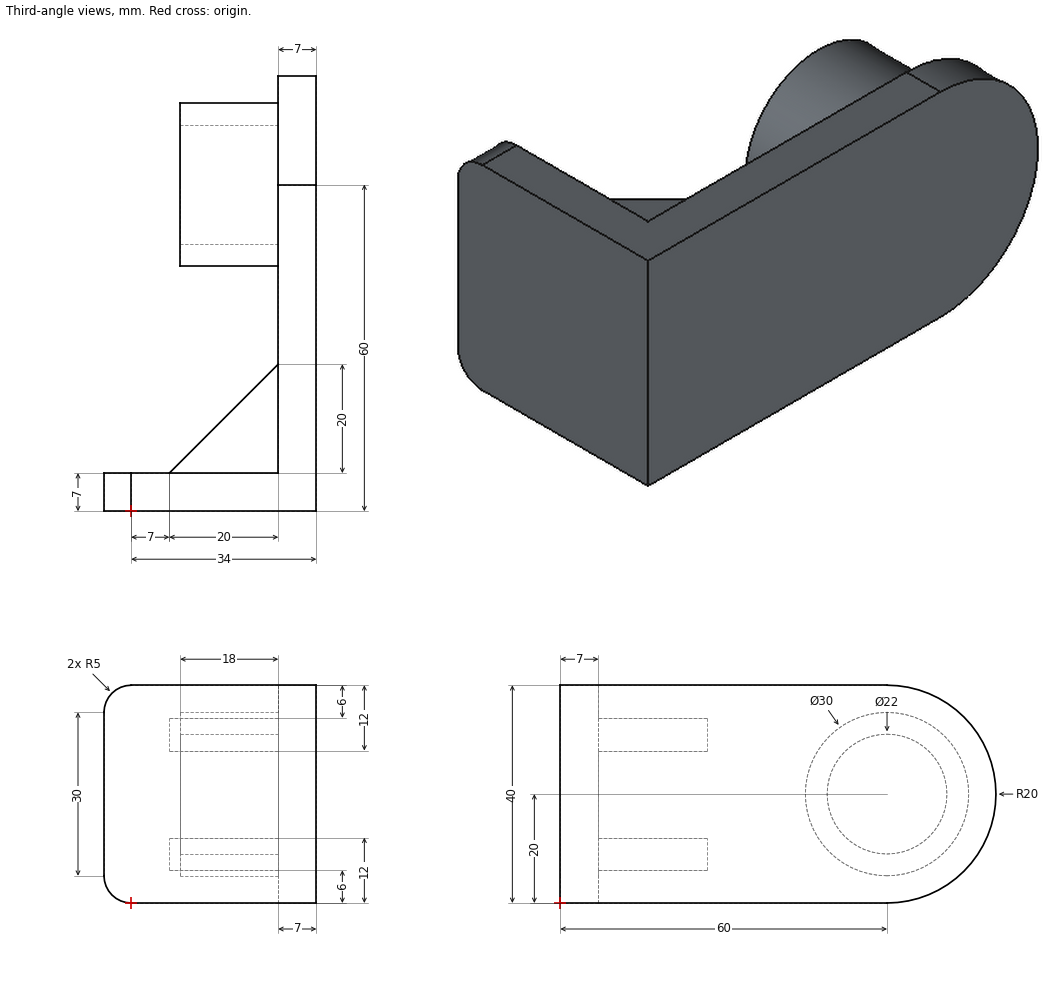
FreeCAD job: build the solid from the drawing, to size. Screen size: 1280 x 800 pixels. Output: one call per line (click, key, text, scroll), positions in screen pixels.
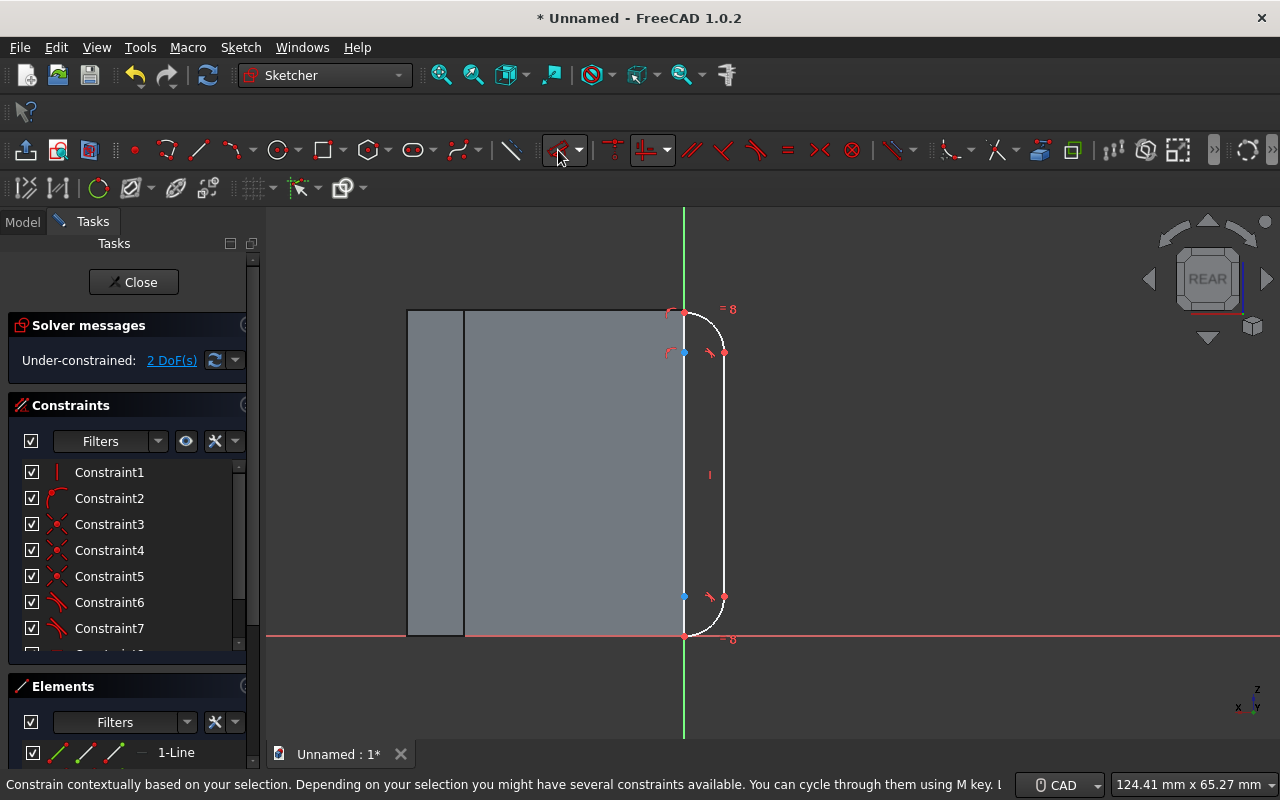
click(720, 334)
click(748, 319)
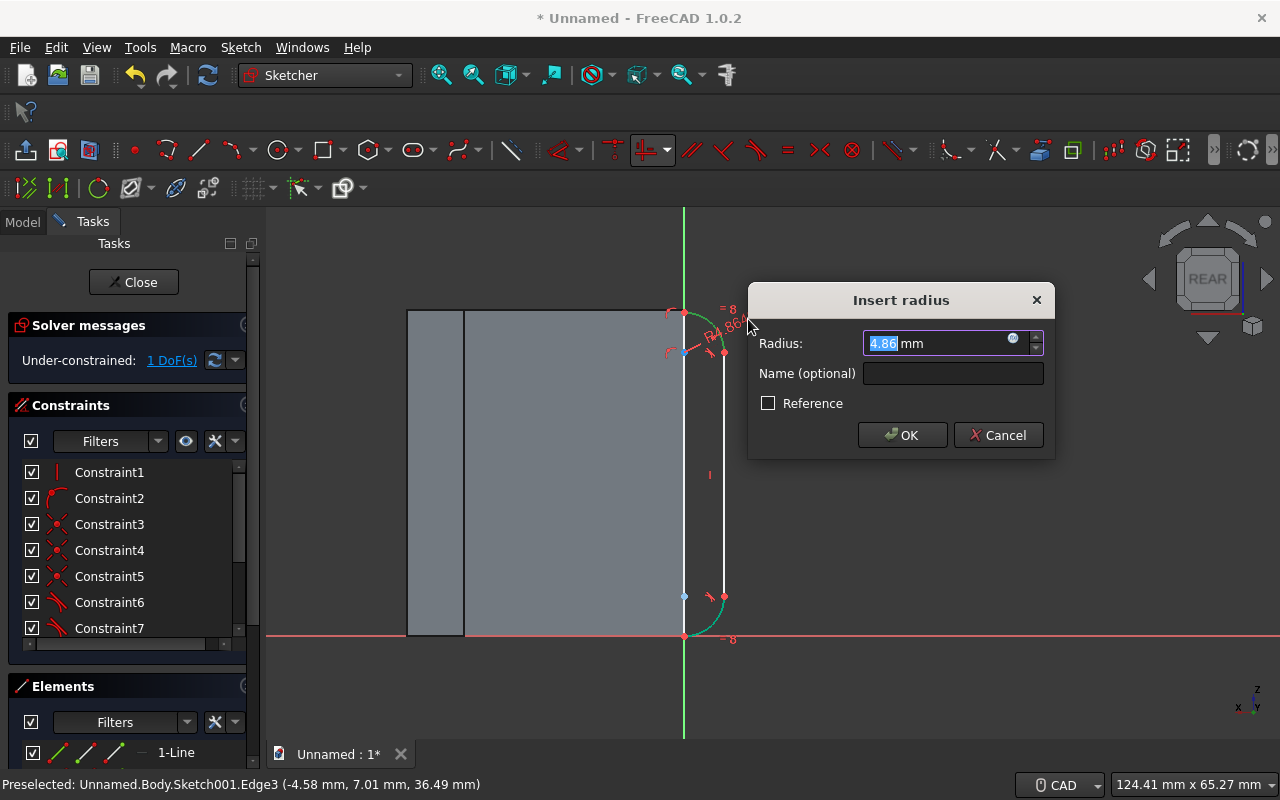
text(5)
key(Return)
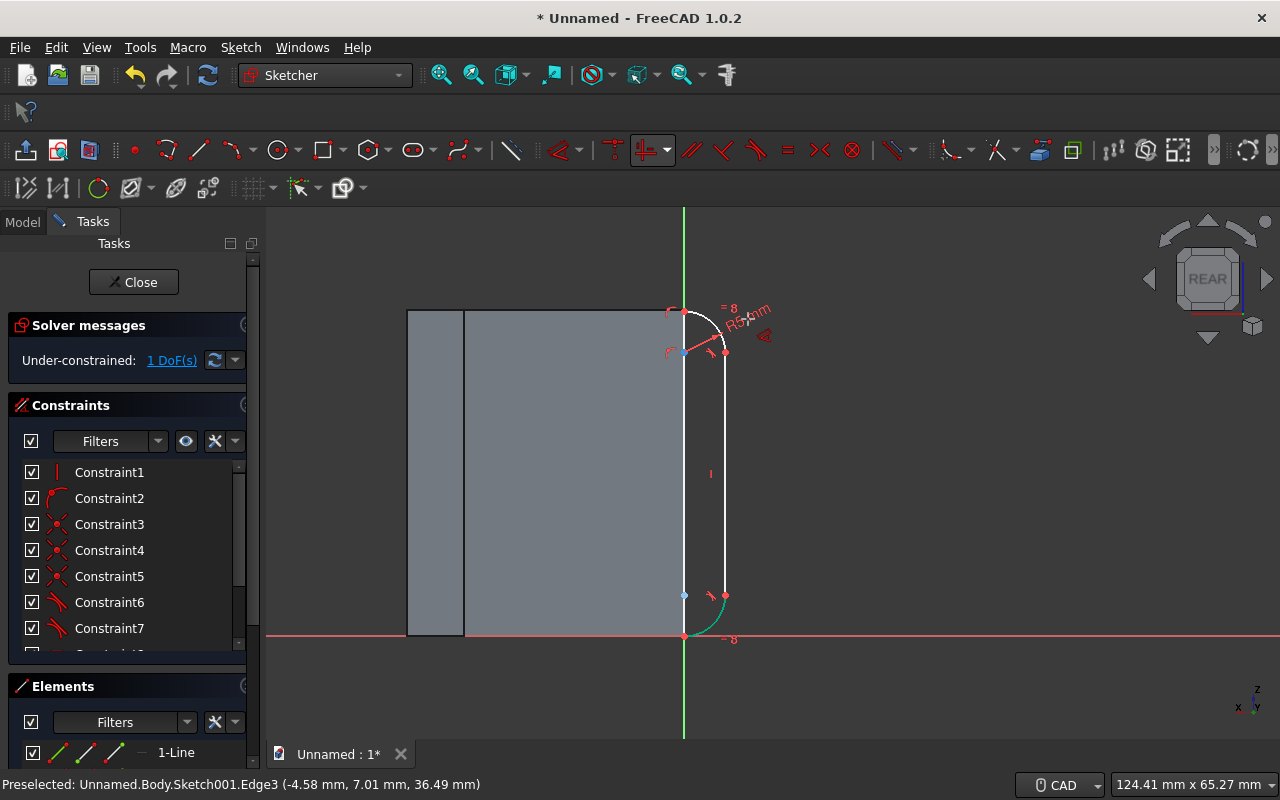
click(725, 523)
click(759, 474)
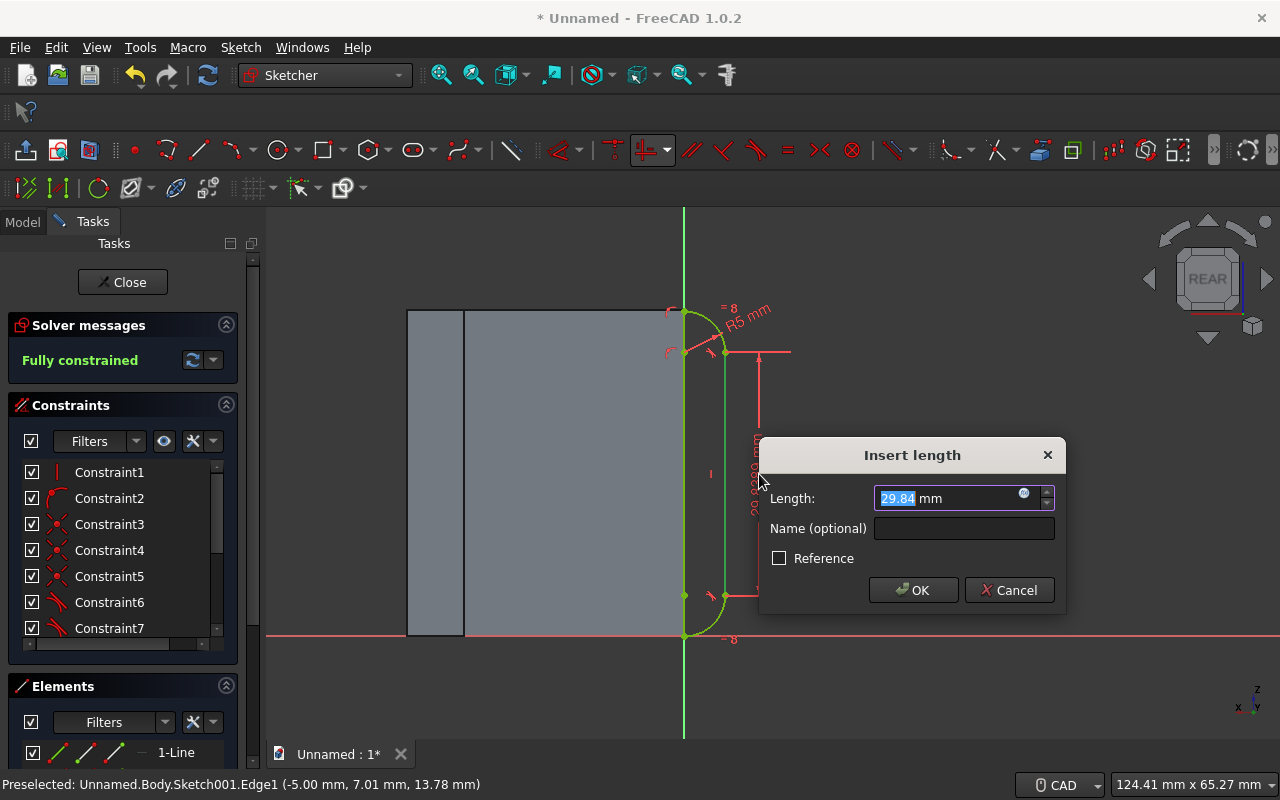
text(30)
key(Return)
key(Escape)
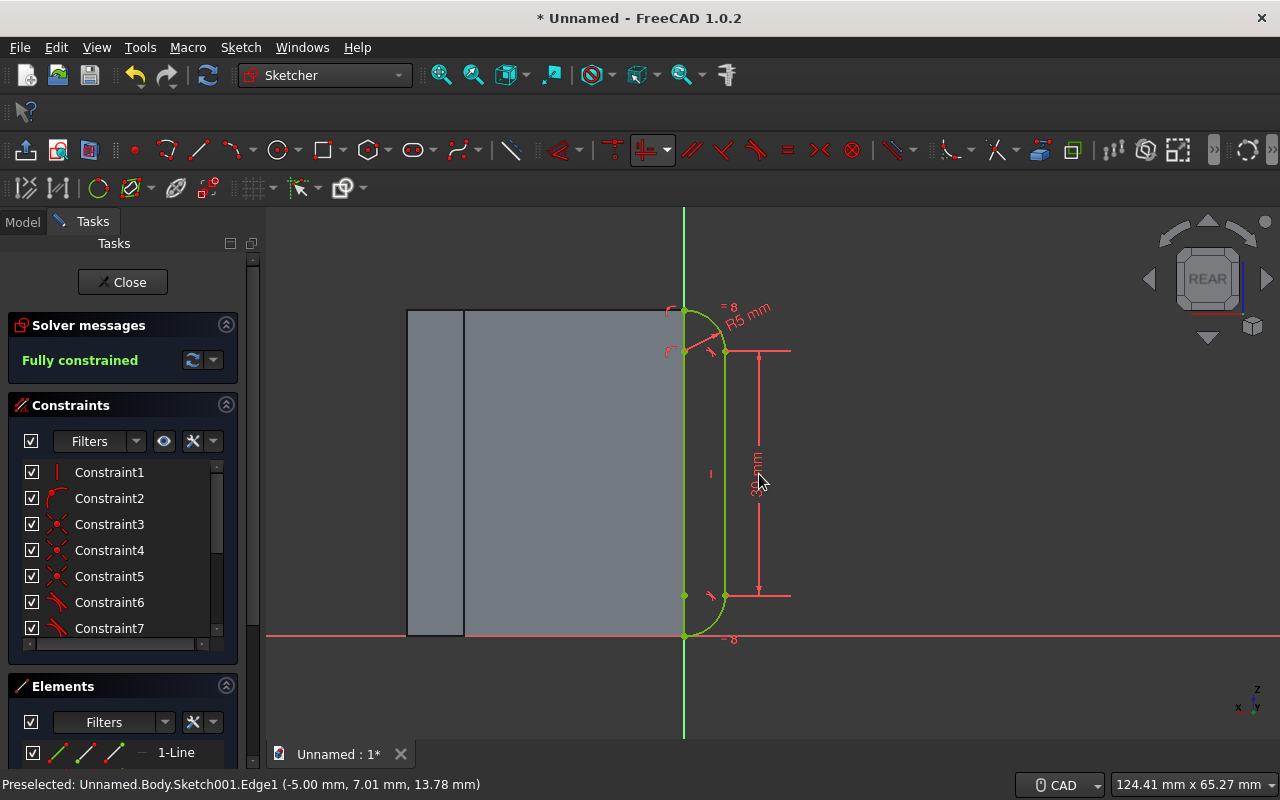
click(123, 282)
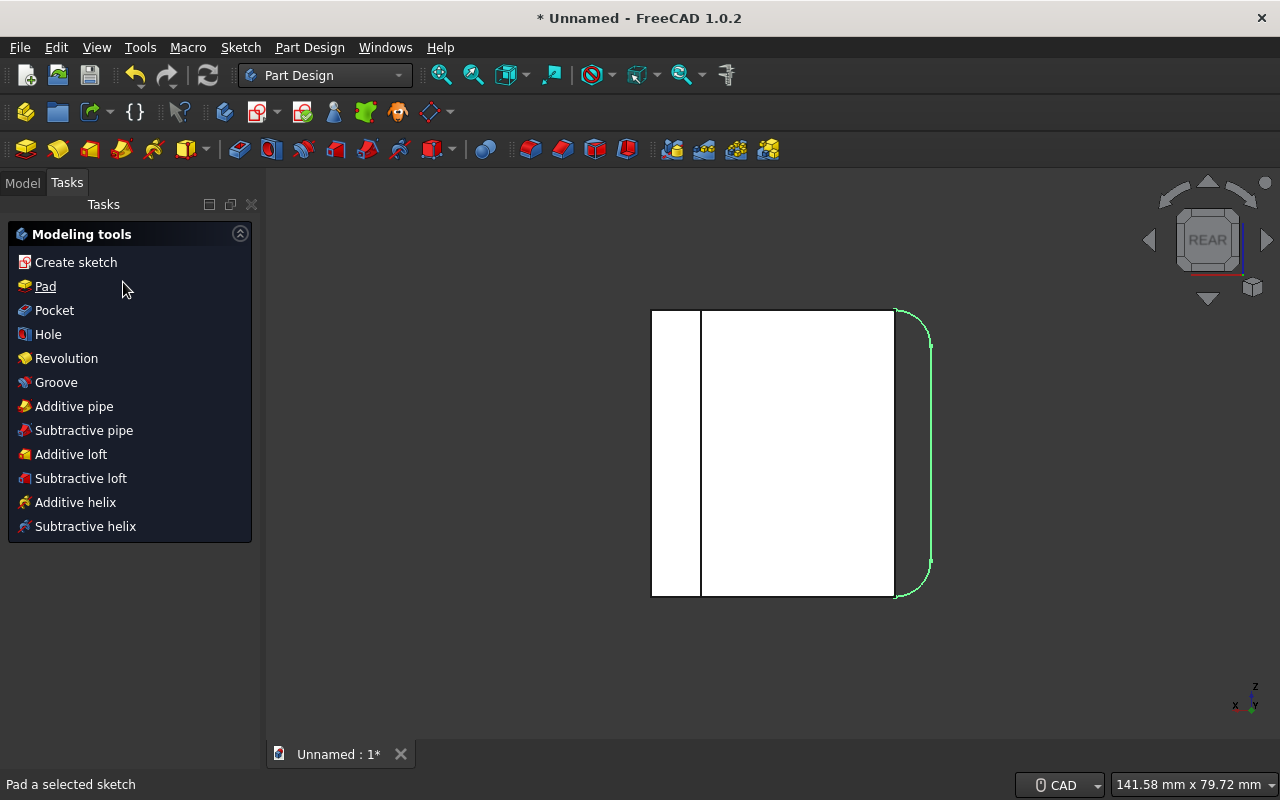
click(26, 150)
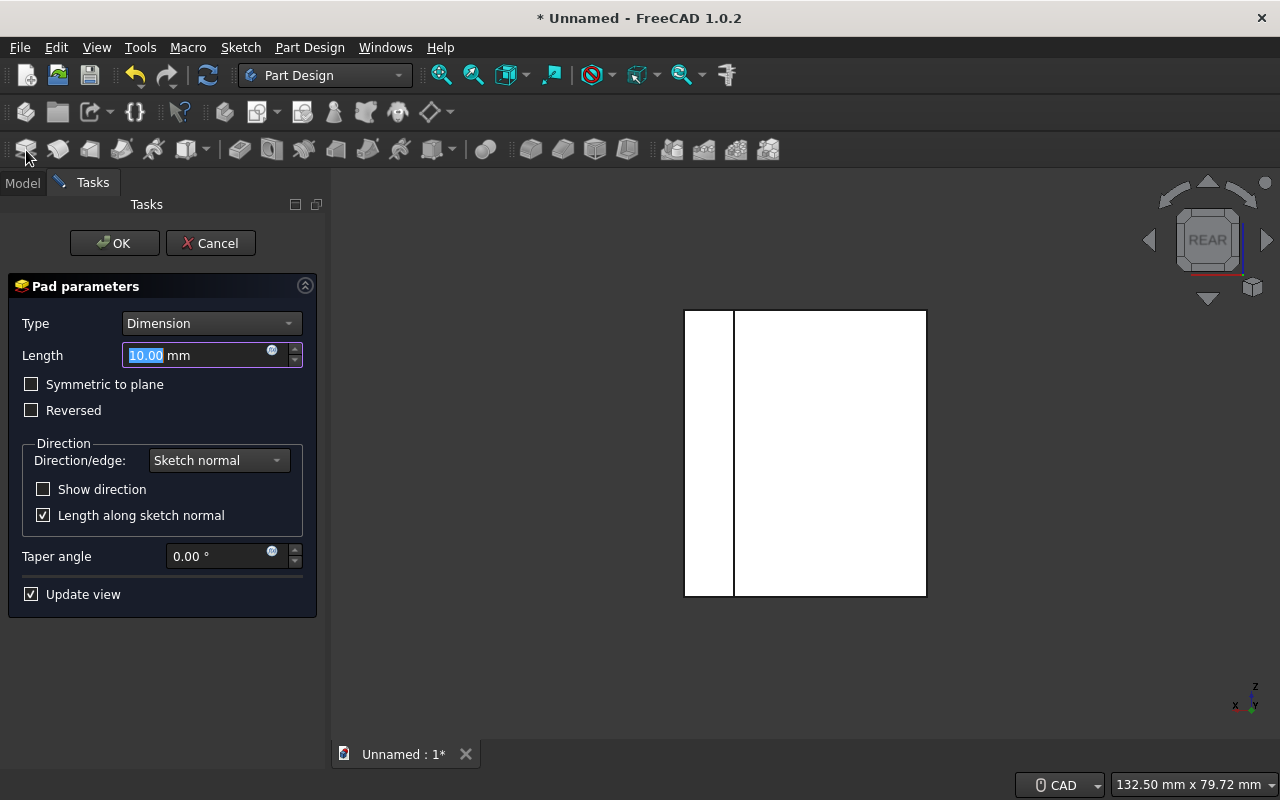
text(7)
key(Tab)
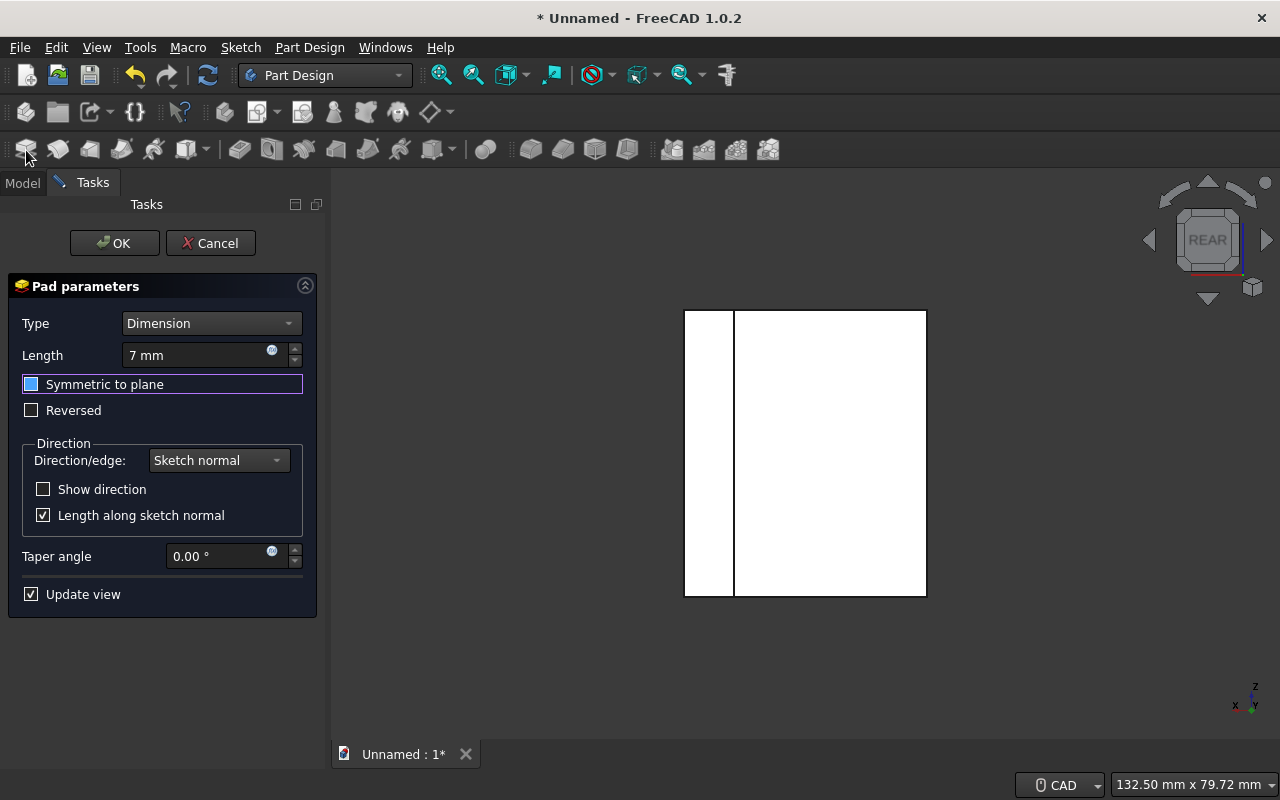
click(30, 410)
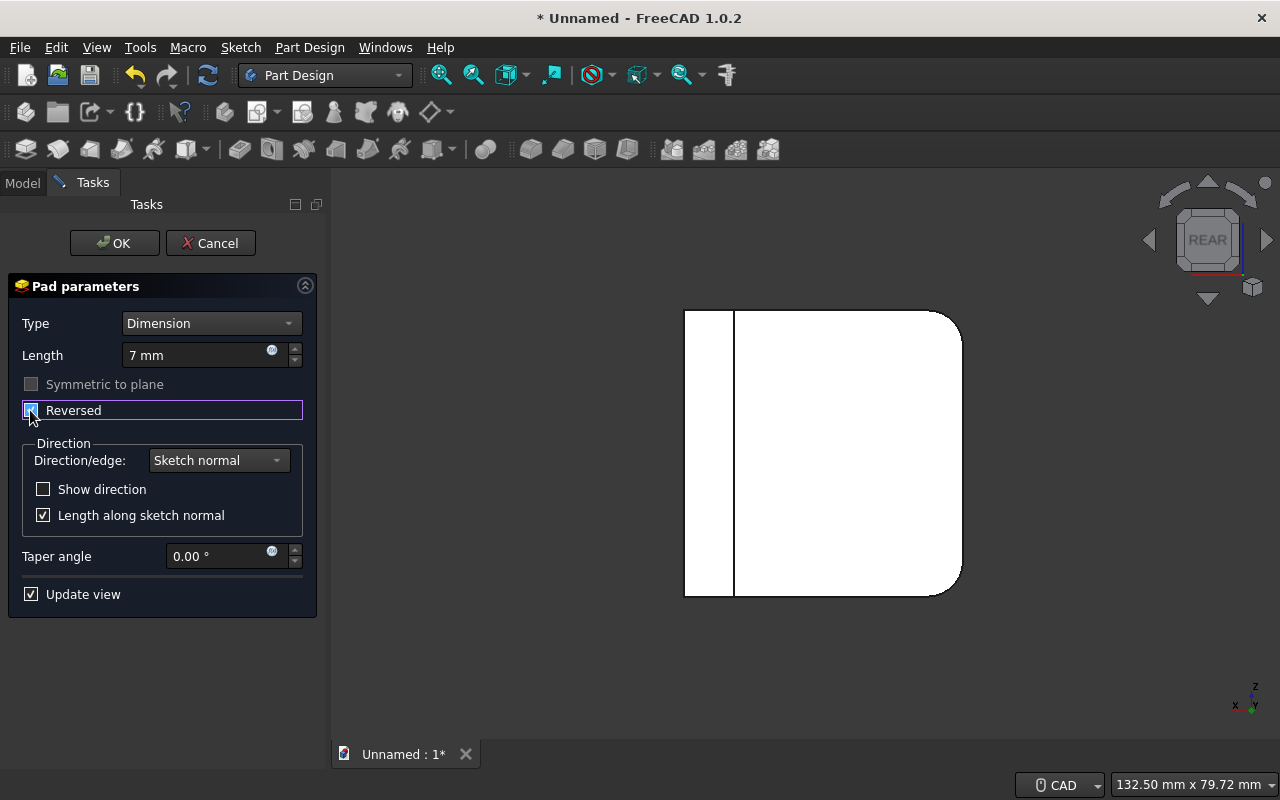
click(115, 243)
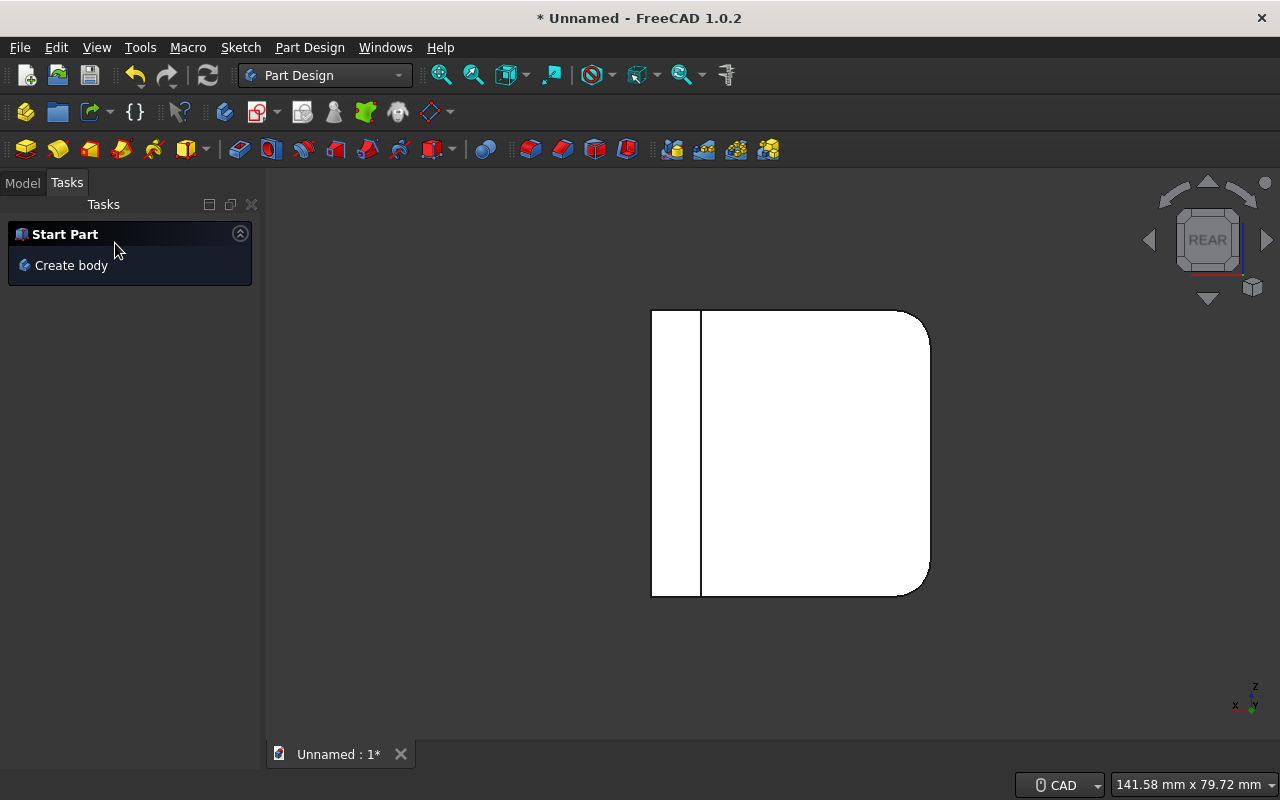
key(6)